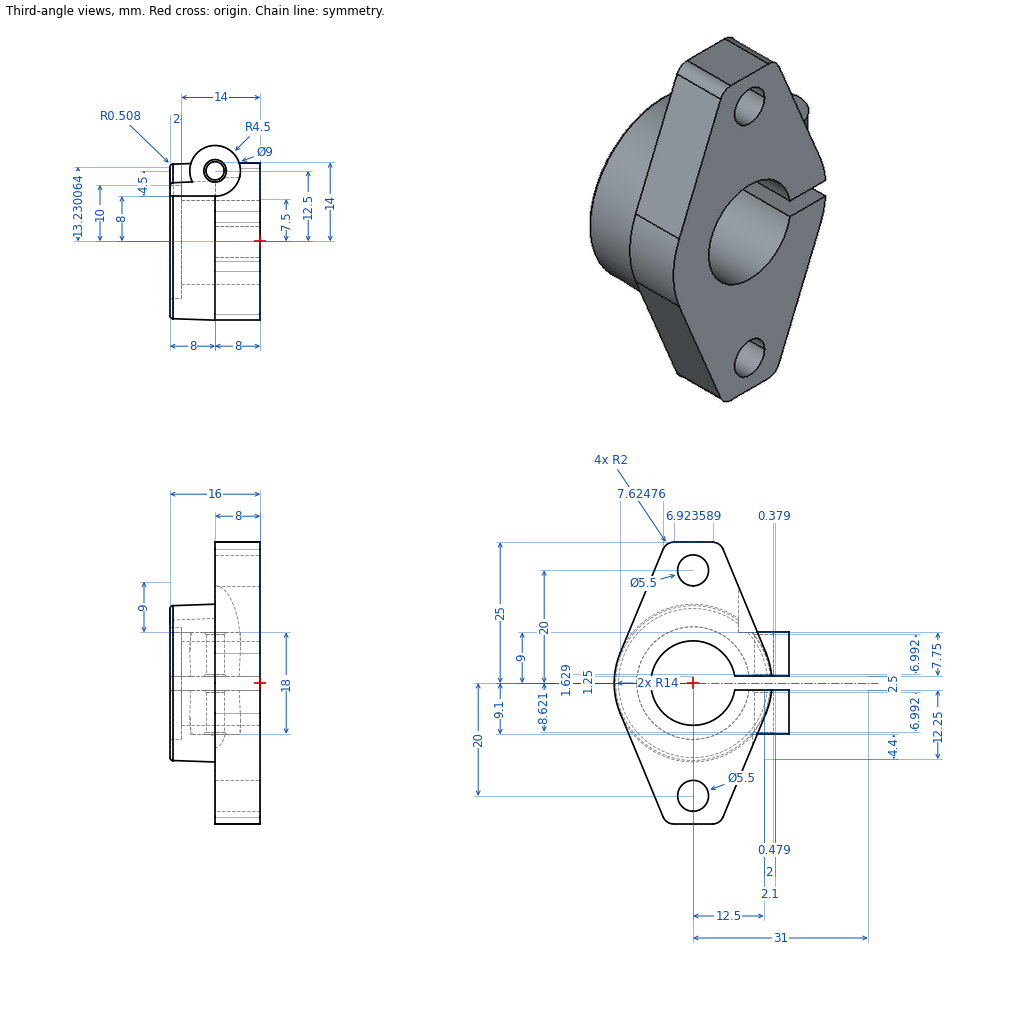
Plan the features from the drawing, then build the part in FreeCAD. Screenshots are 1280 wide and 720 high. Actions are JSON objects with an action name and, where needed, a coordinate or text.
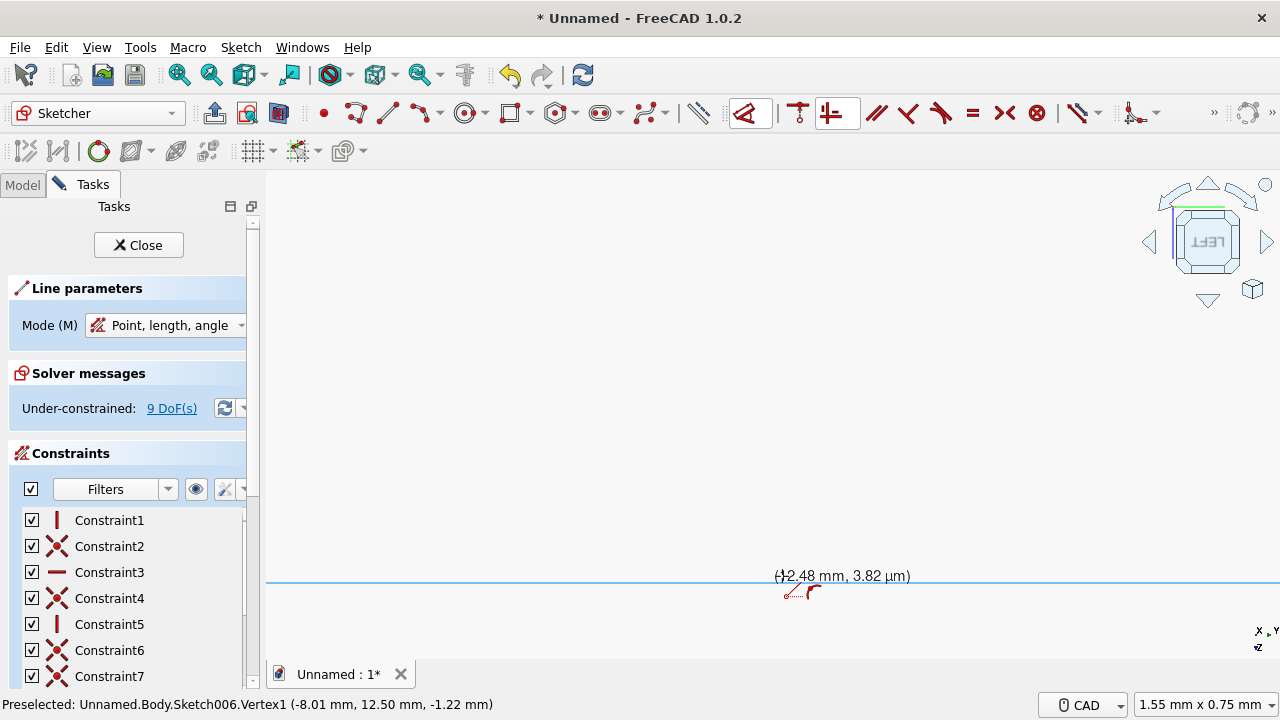
{"action": "left_click", "coordinate": [781, 567]}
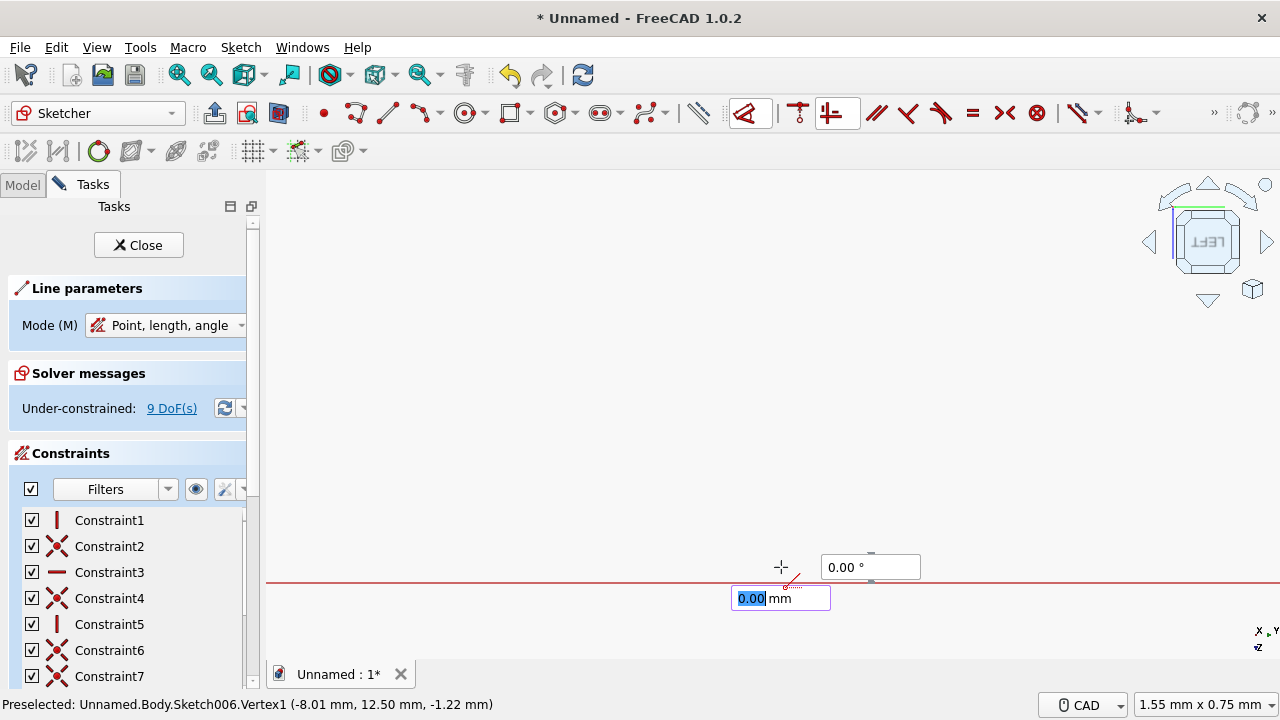
{"action": "scroll", "coordinate": [819, 520], "scroll_direction": "down", "scroll_amount": 17}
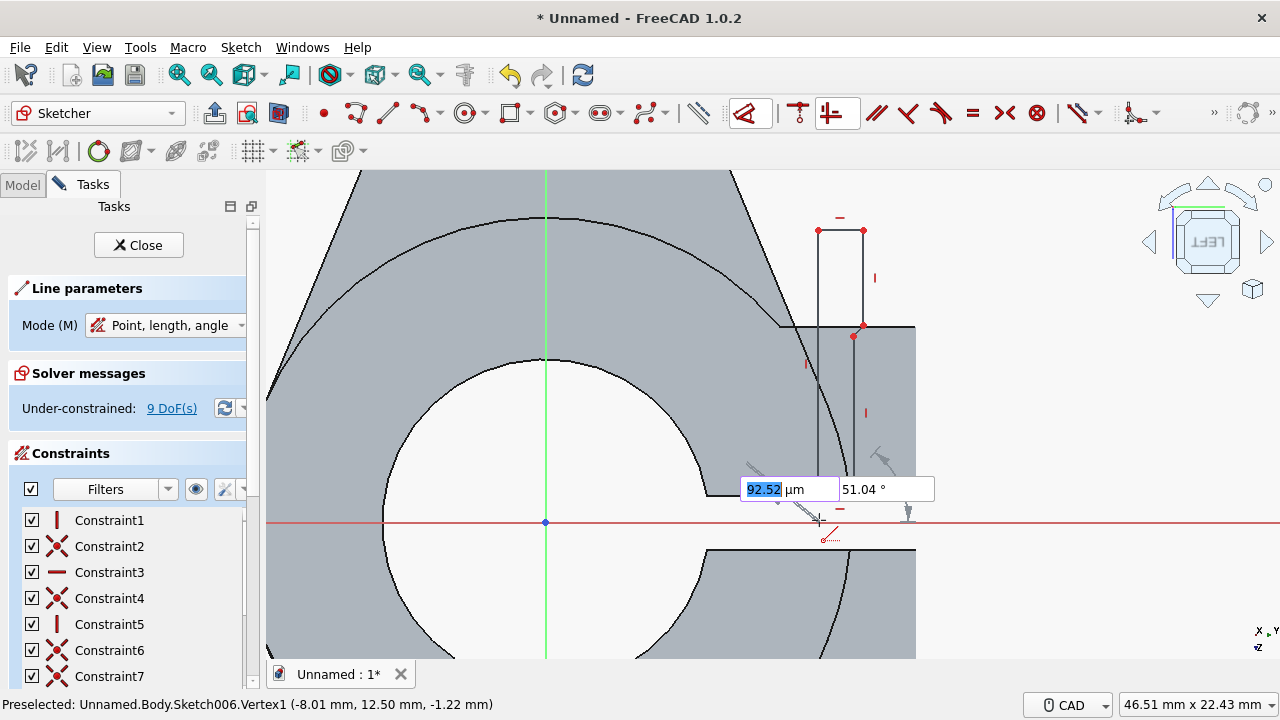
{"action": "left_click", "coordinate": [818, 602]}
{"action": "key", "text": "Escape"}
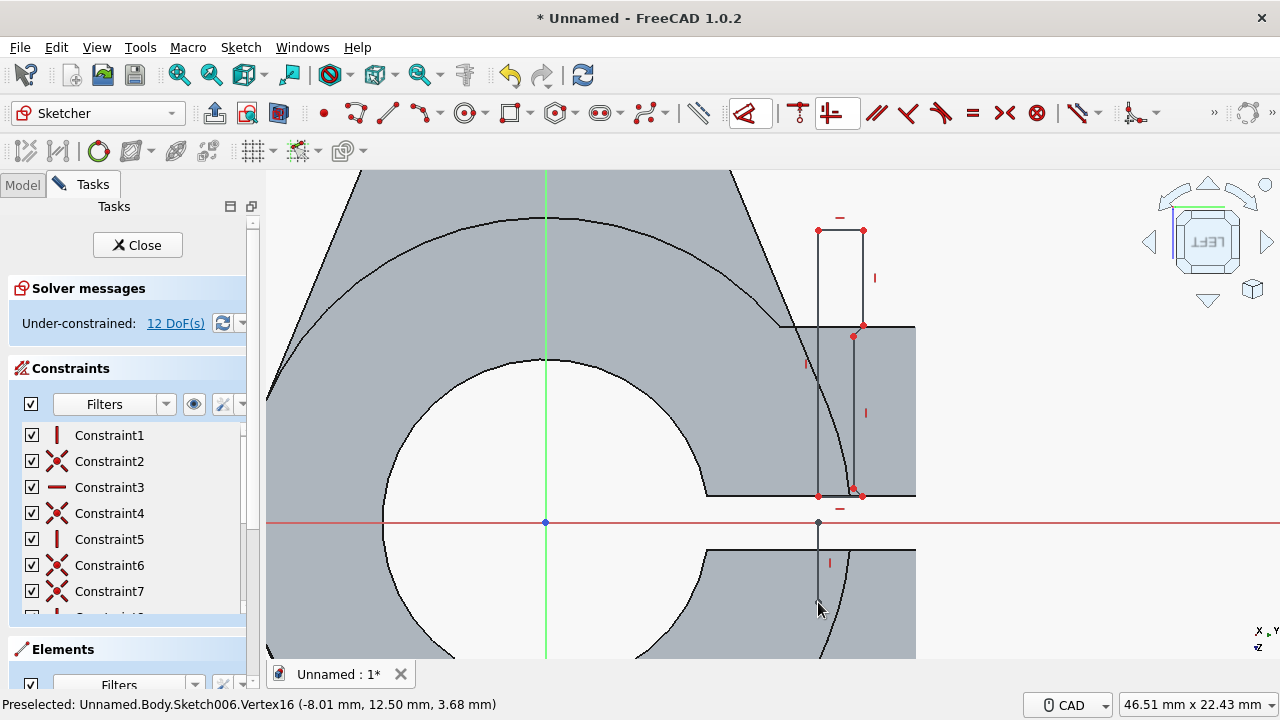
{"action": "left_click", "coordinate": [818, 547]}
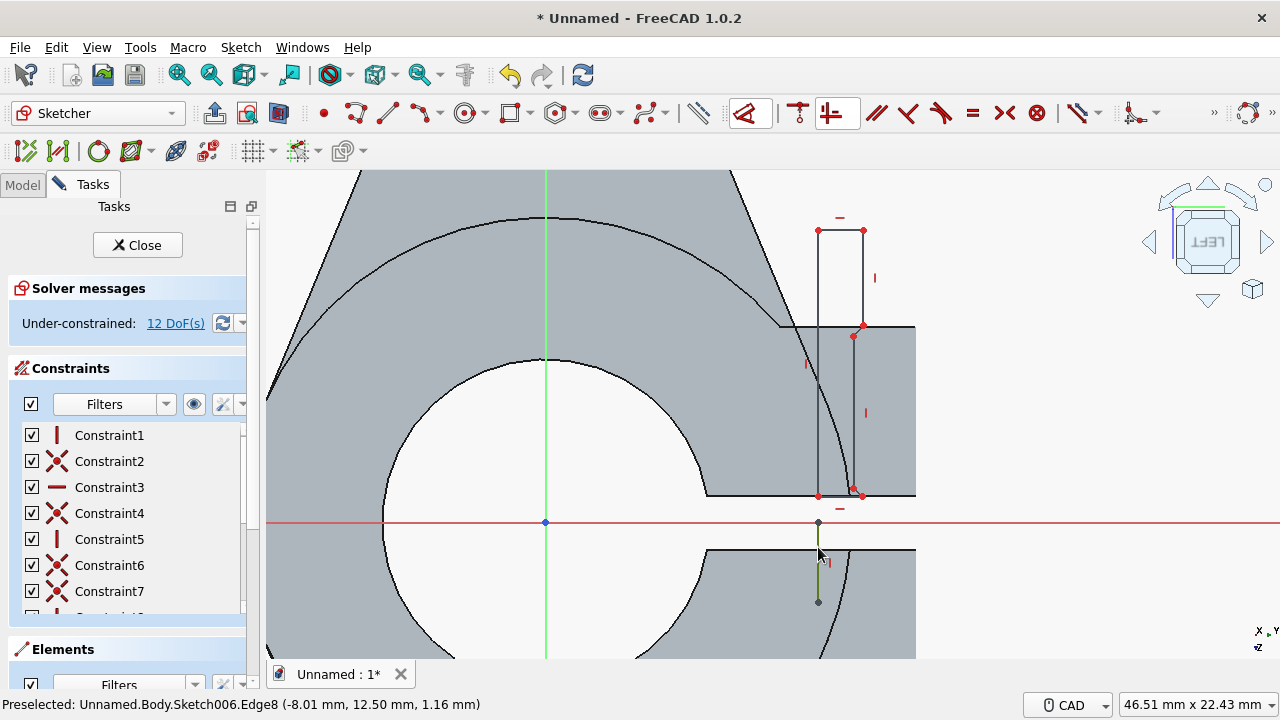
{"action": "left_click", "coordinate": [700, 114]}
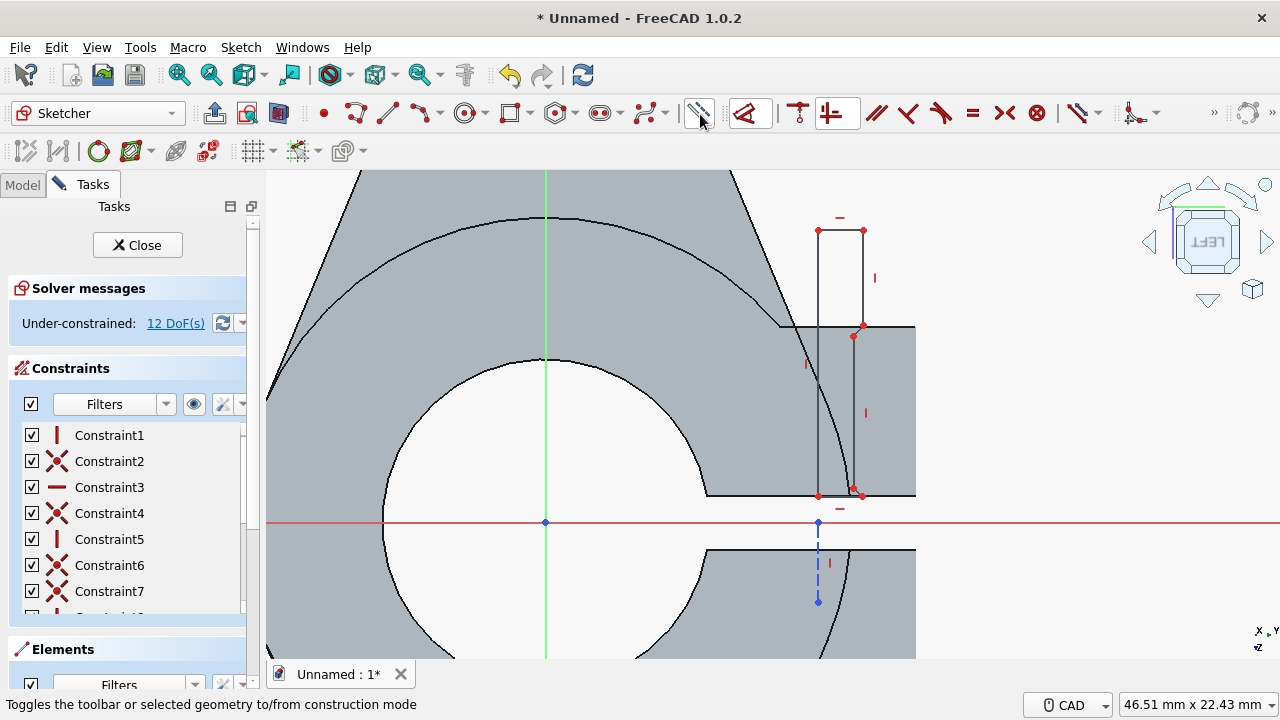
{"action": "scroll", "coordinate": [849, 497], "scroll_direction": "up", "scroll_amount": 2}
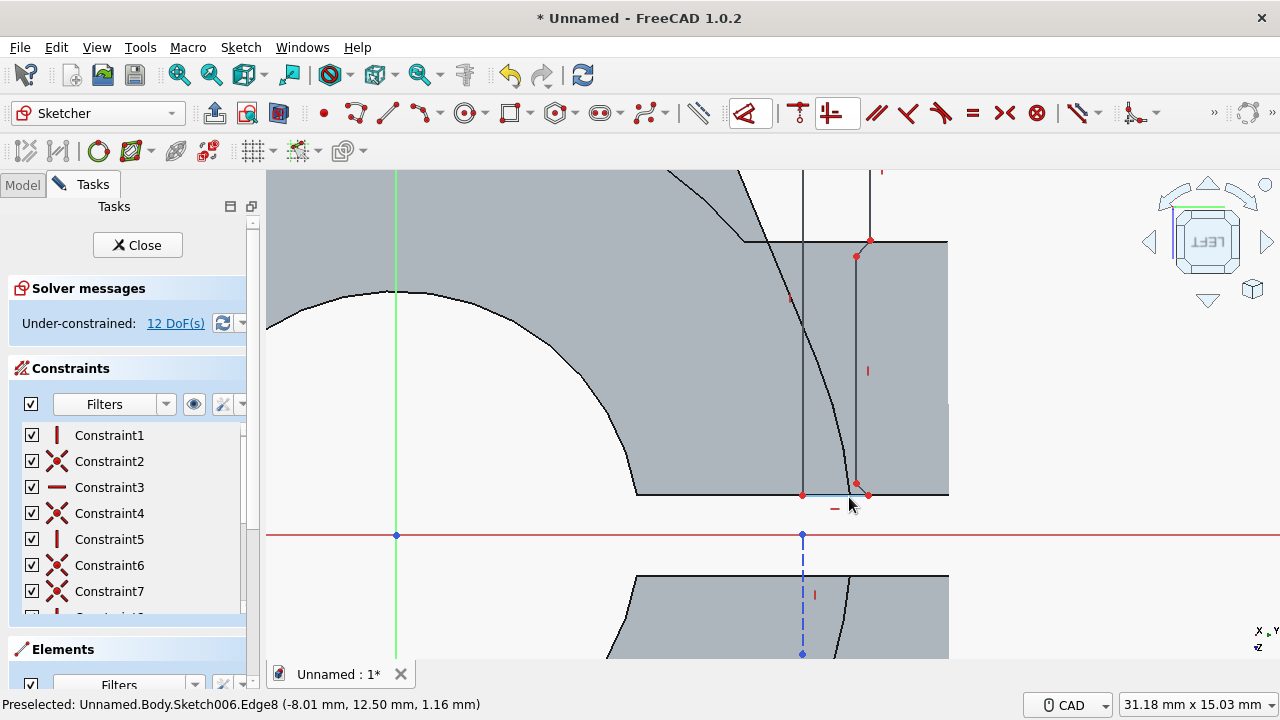
{"action": "left_click", "coordinate": [849, 496]}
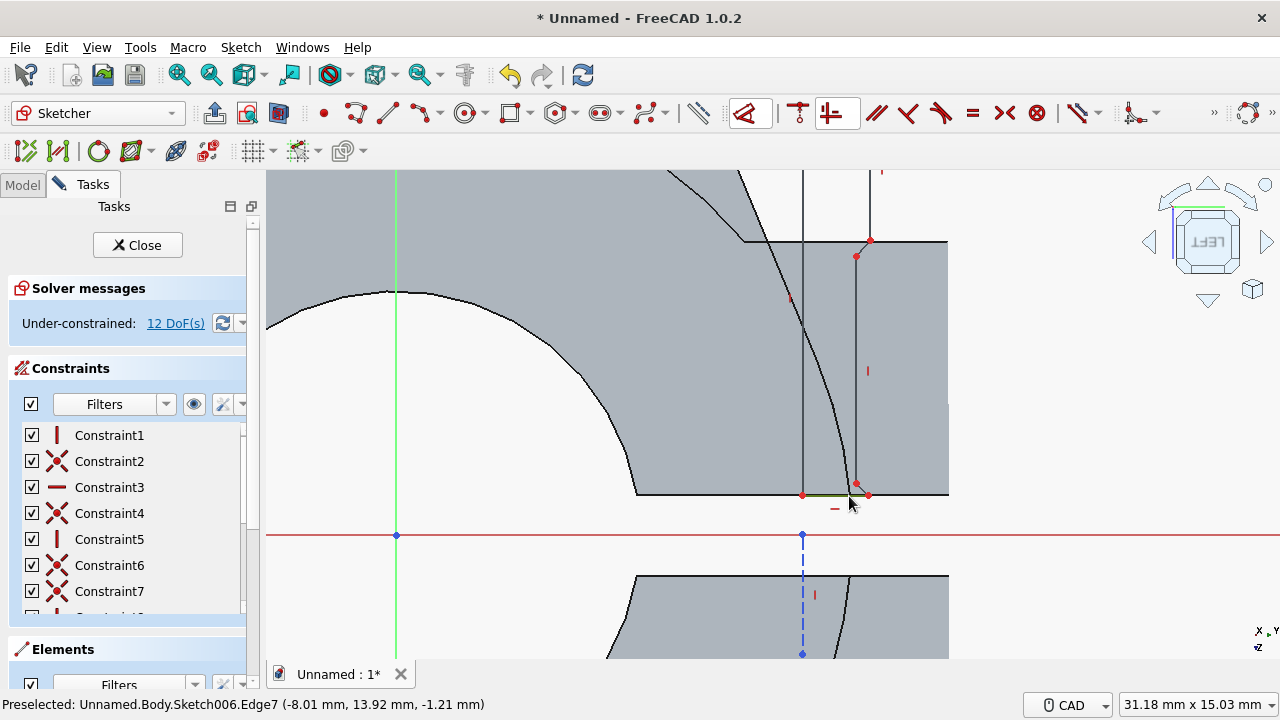
{"action": "key", "text": "l"}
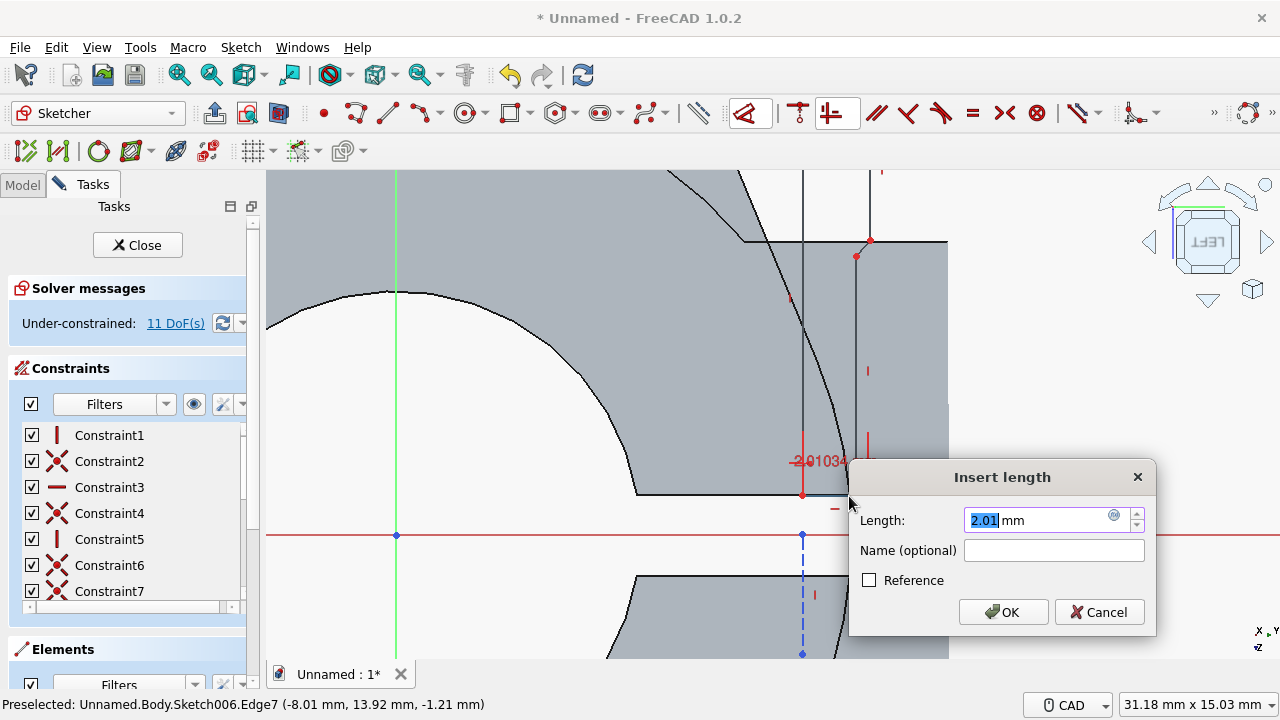
{"action": "type", "text": "2"}
{"action": "key", "text": "Return"}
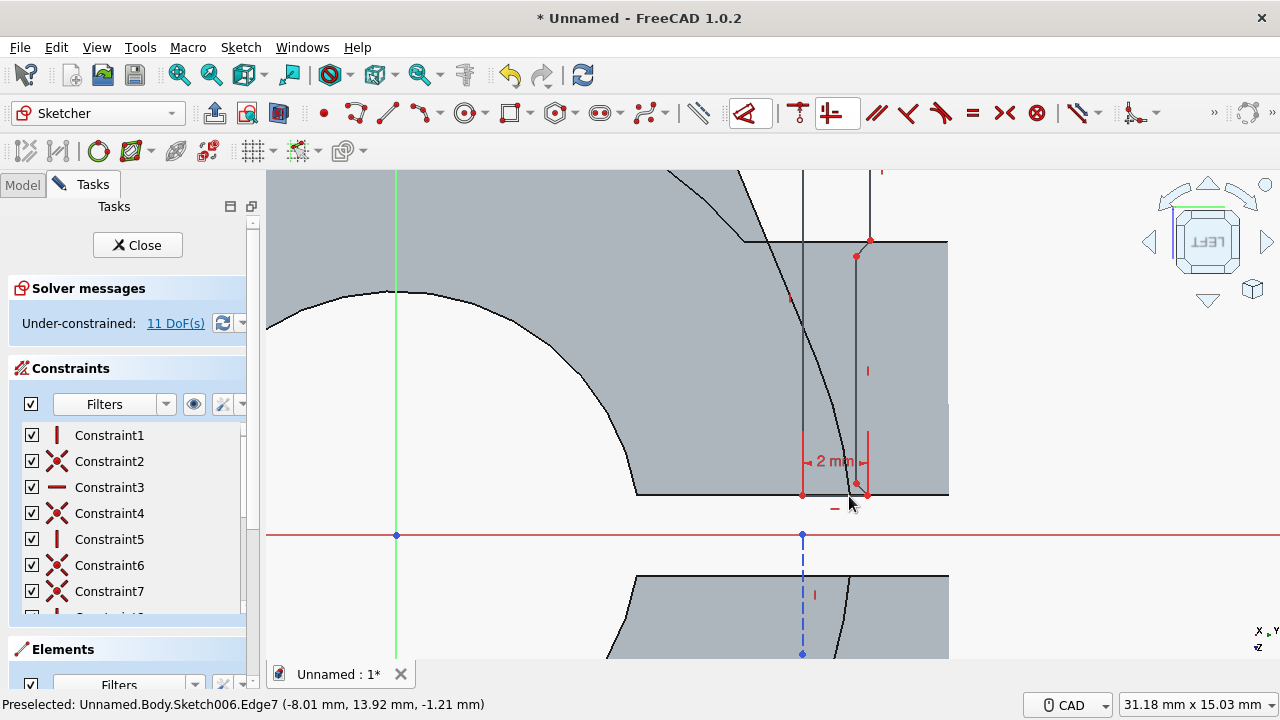
{"action": "scroll", "coordinate": [791, 463], "scroll_direction": "down", "scroll_amount": 3}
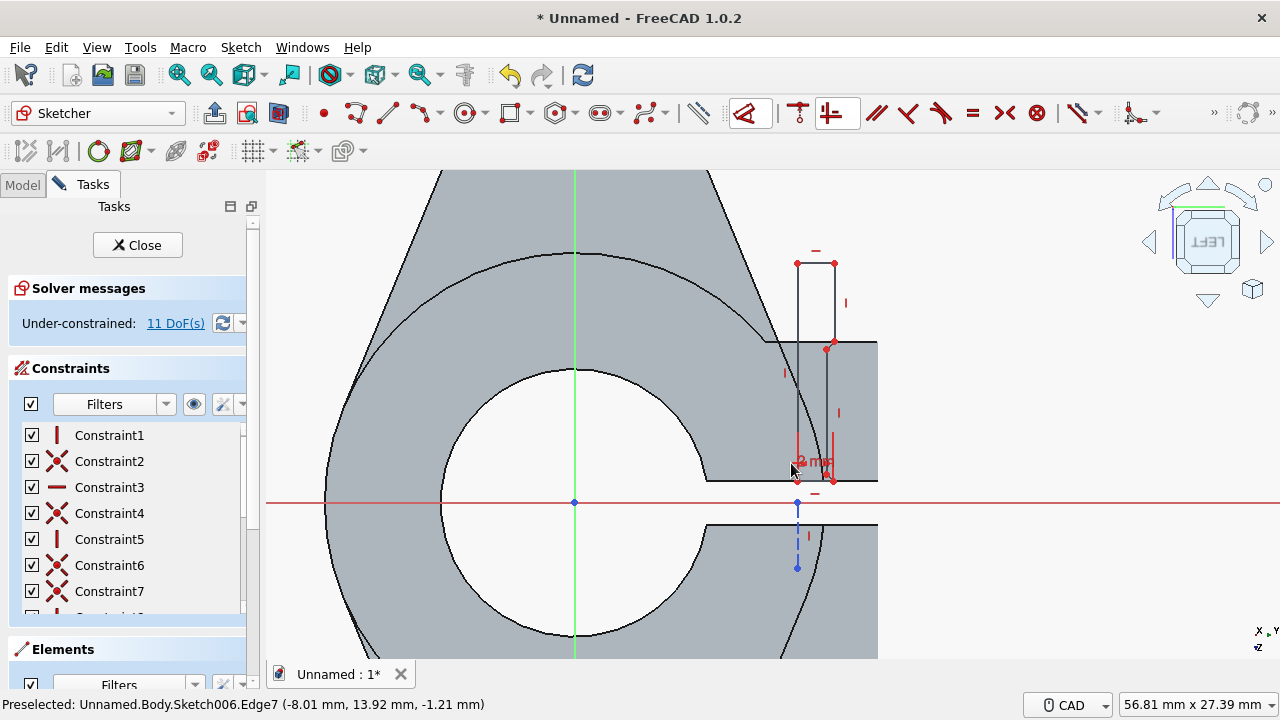
{"action": "scroll", "coordinate": [809, 263], "scroll_direction": "up", "scroll_amount": 2}